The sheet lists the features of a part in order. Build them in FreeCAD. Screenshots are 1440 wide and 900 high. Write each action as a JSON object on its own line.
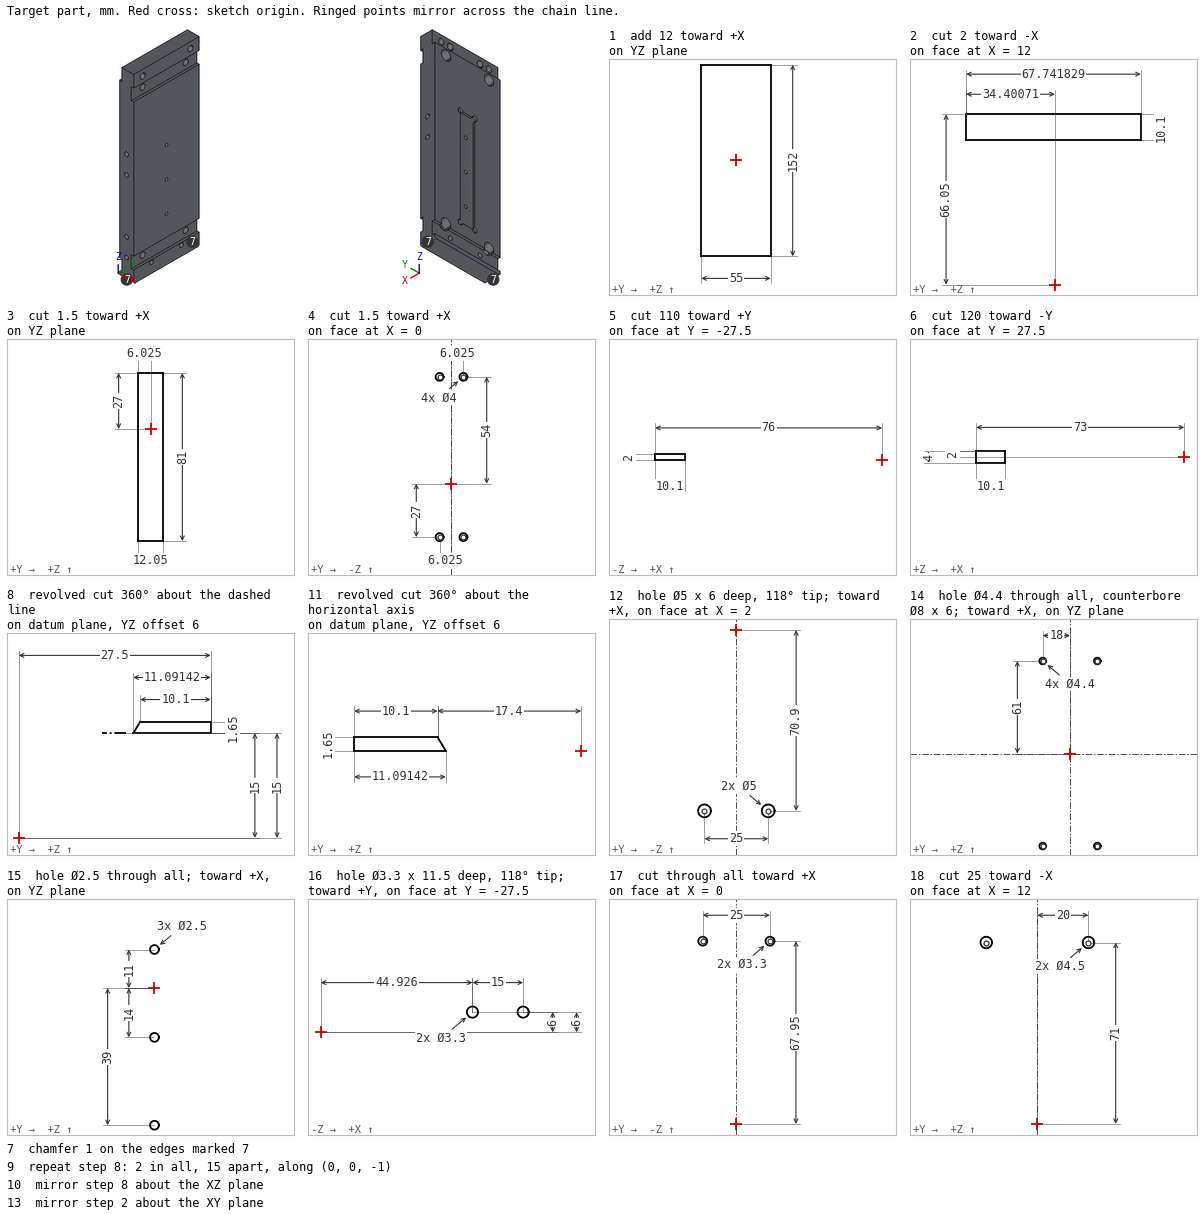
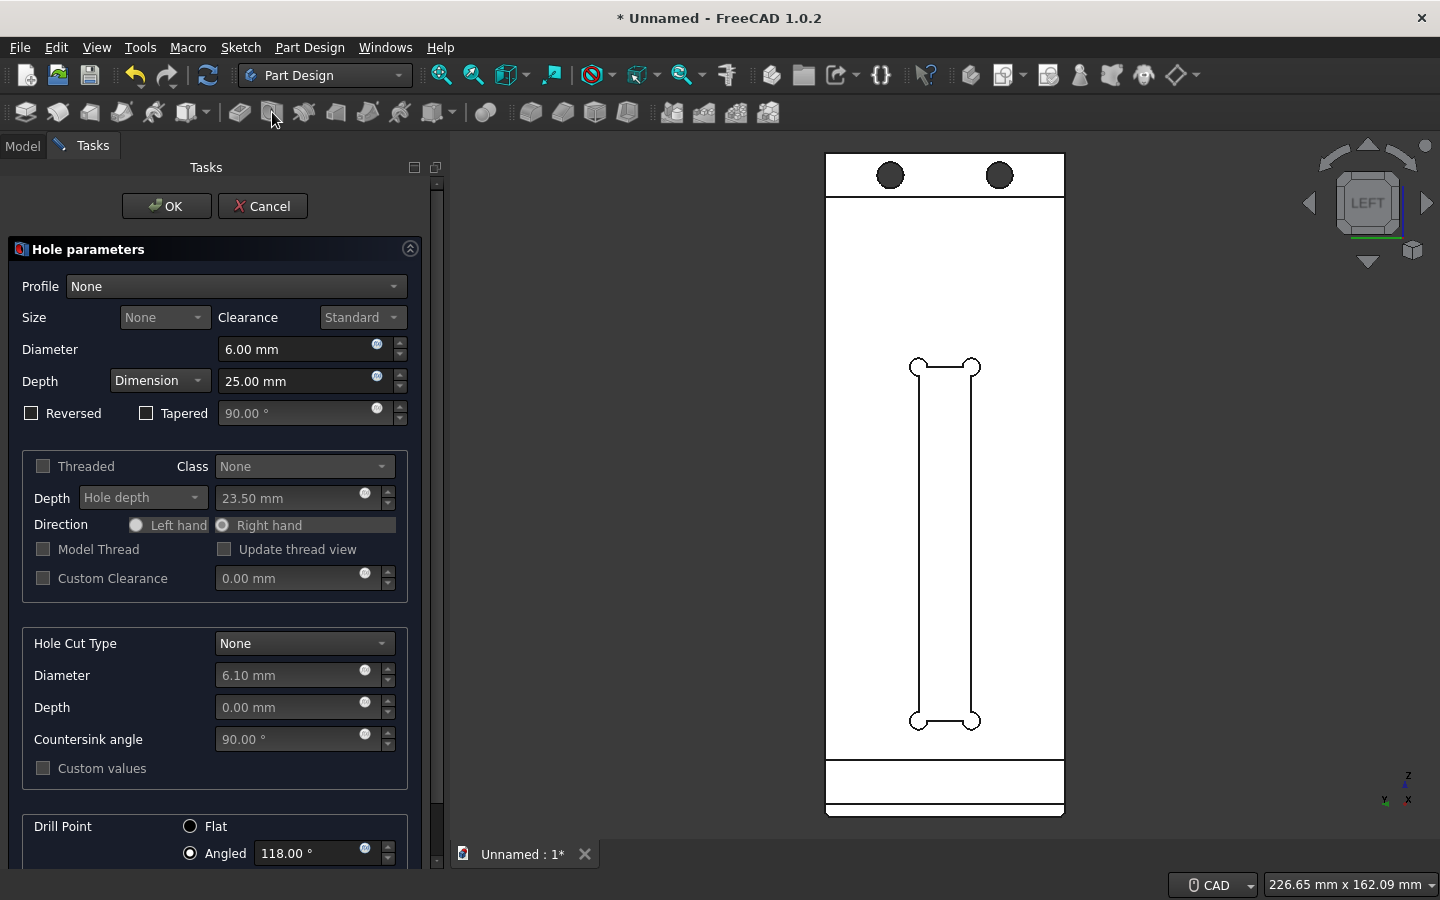
{"action": "triple_click", "coordinate": [305, 349]}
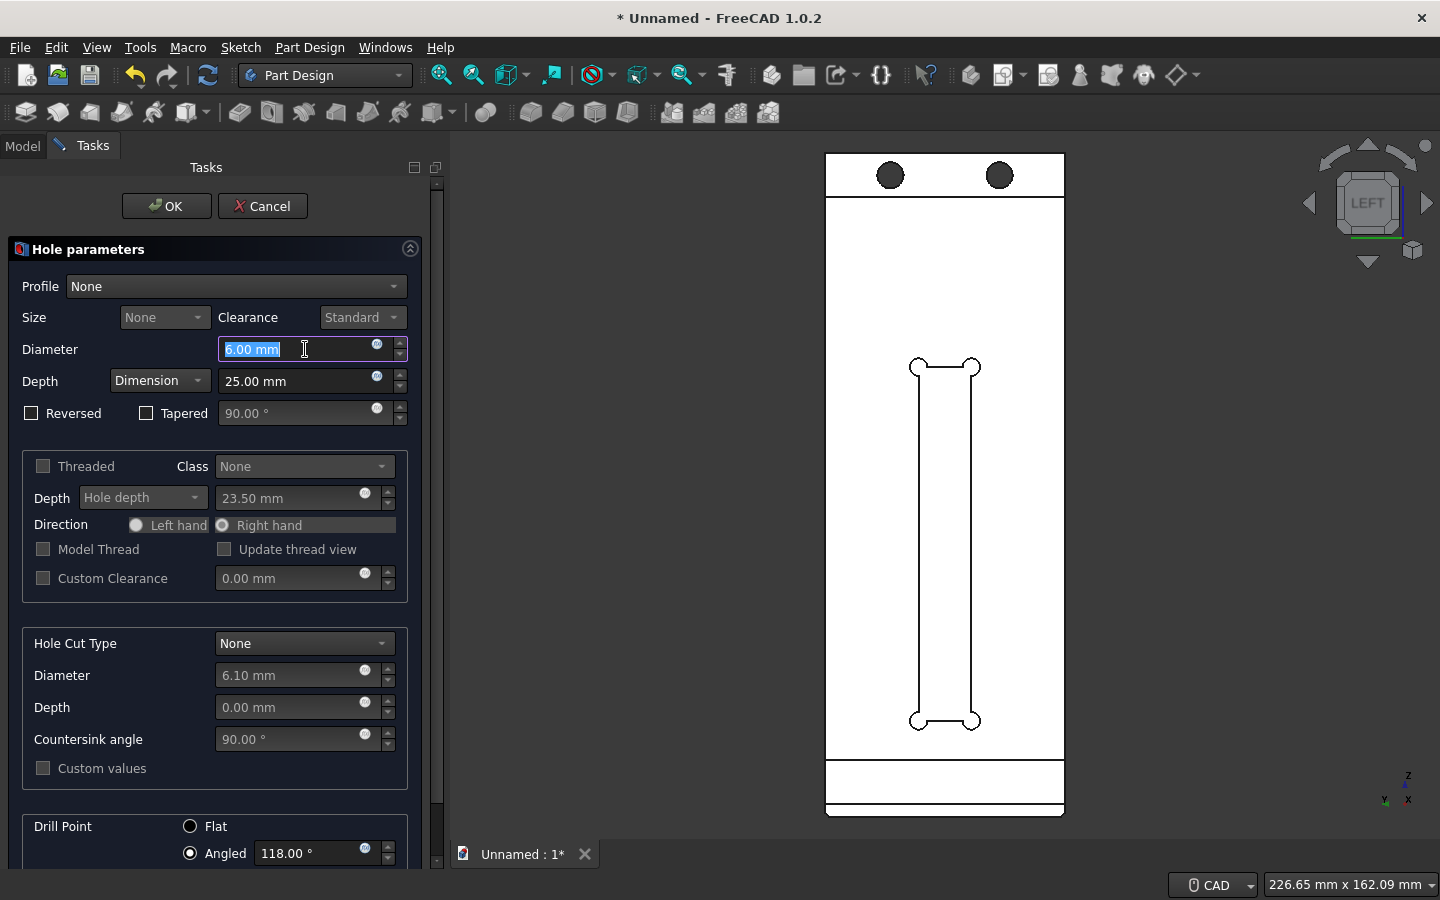
{"action": "type", "text": "5"}
{"action": "key", "text": "Tab"}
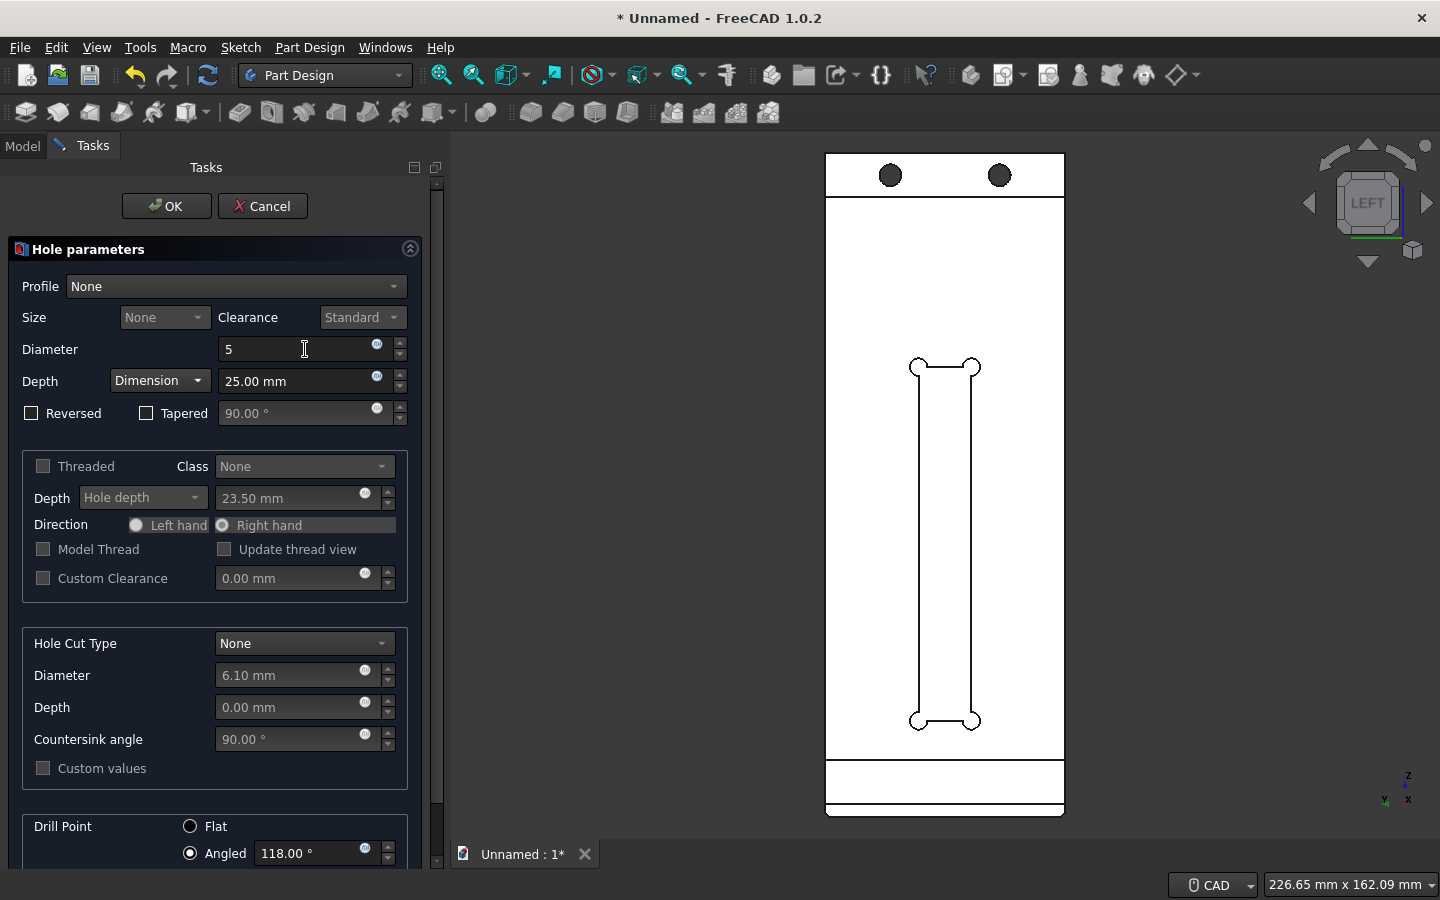
{"action": "triple_click", "coordinate": [305, 381]}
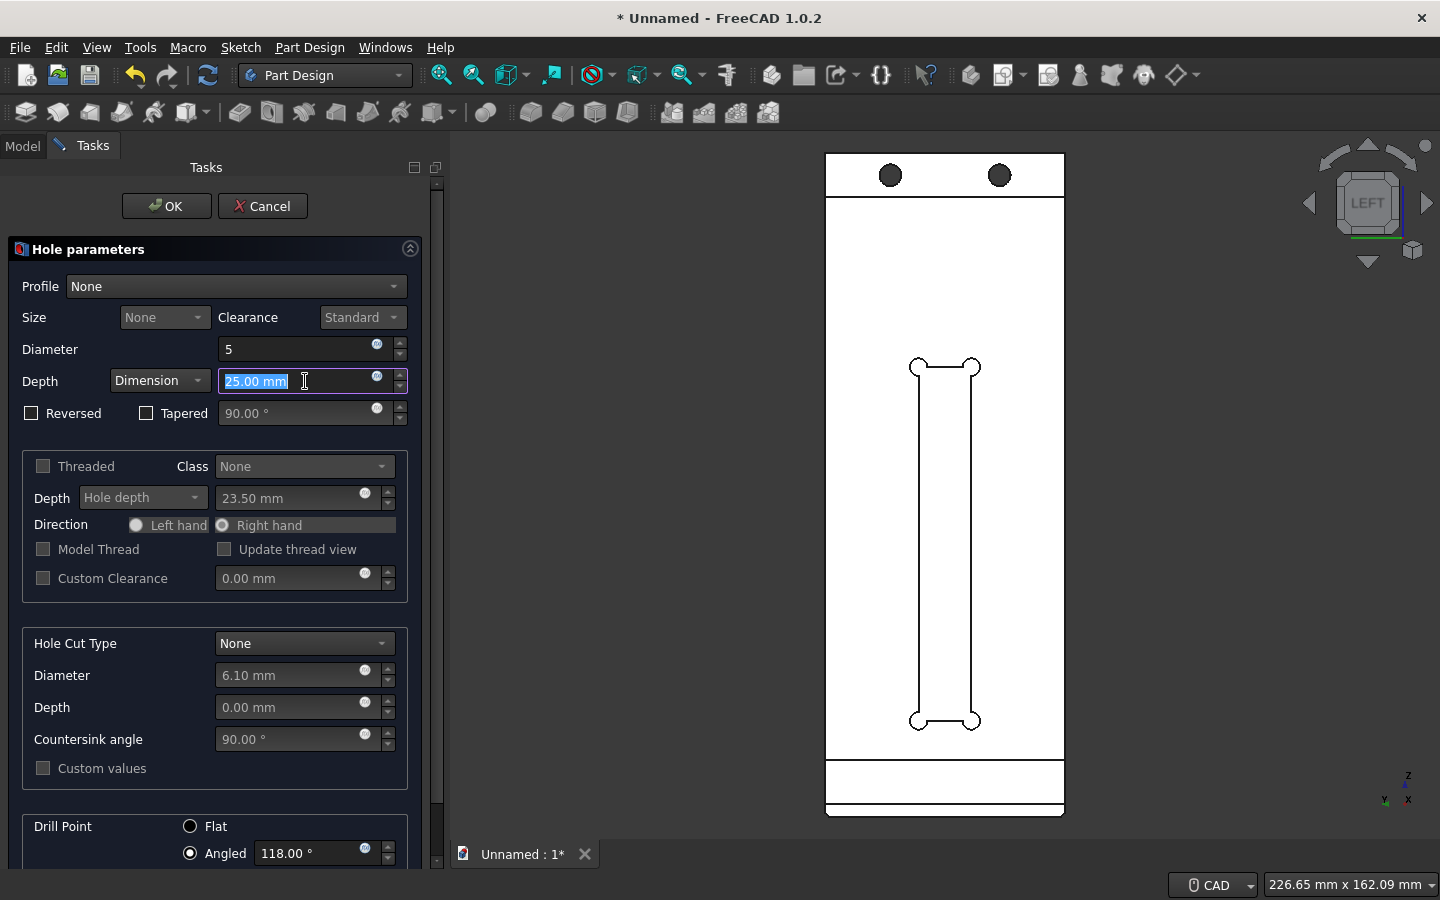
{"action": "type", "text": "6"}
{"action": "key", "text": "Tab"}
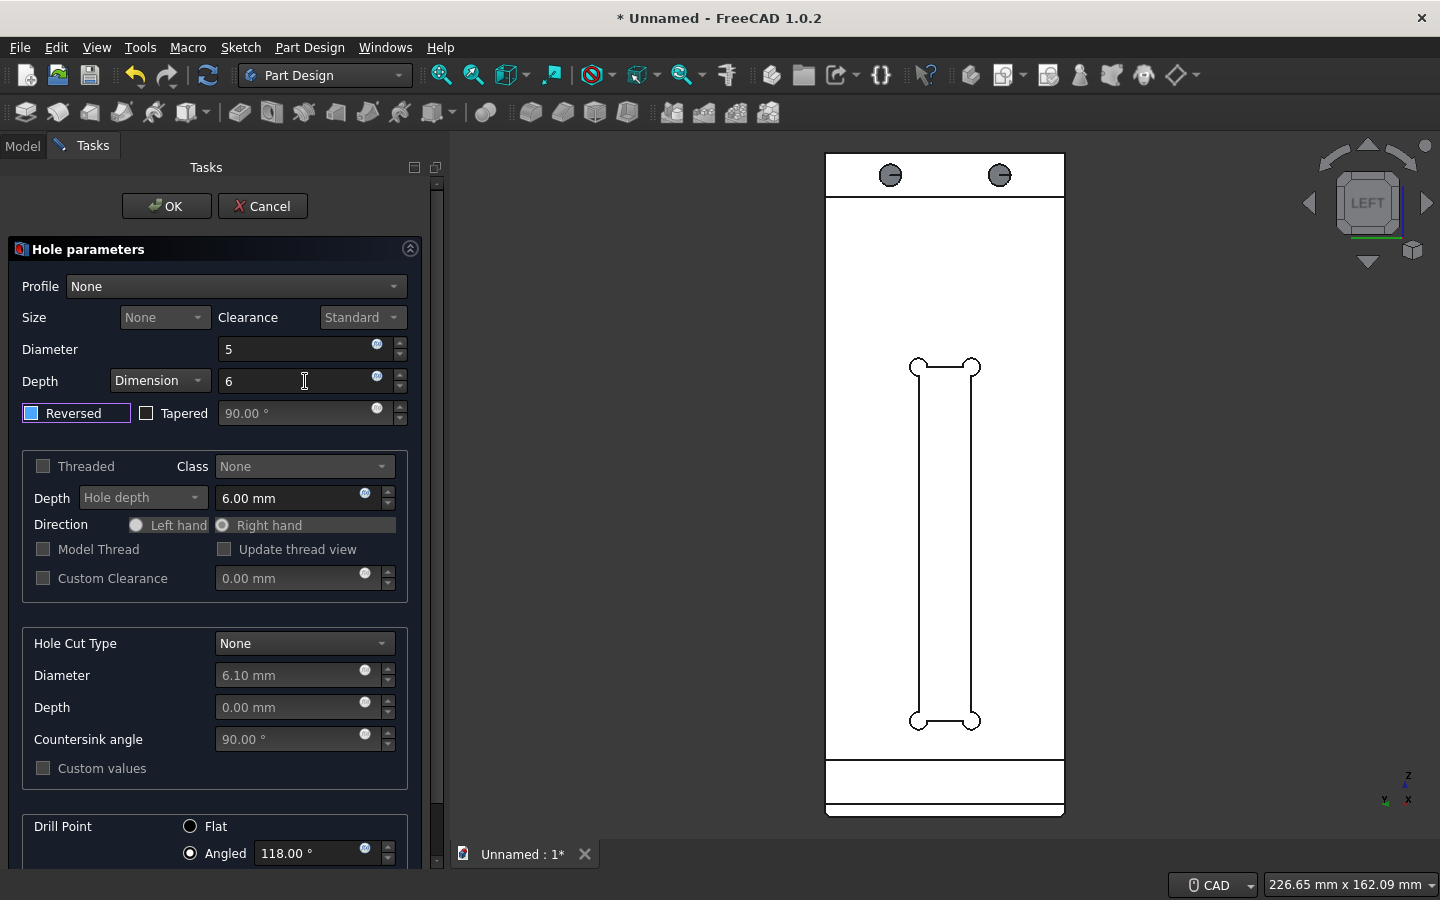
{"action": "left_click", "coordinate": [167, 206]}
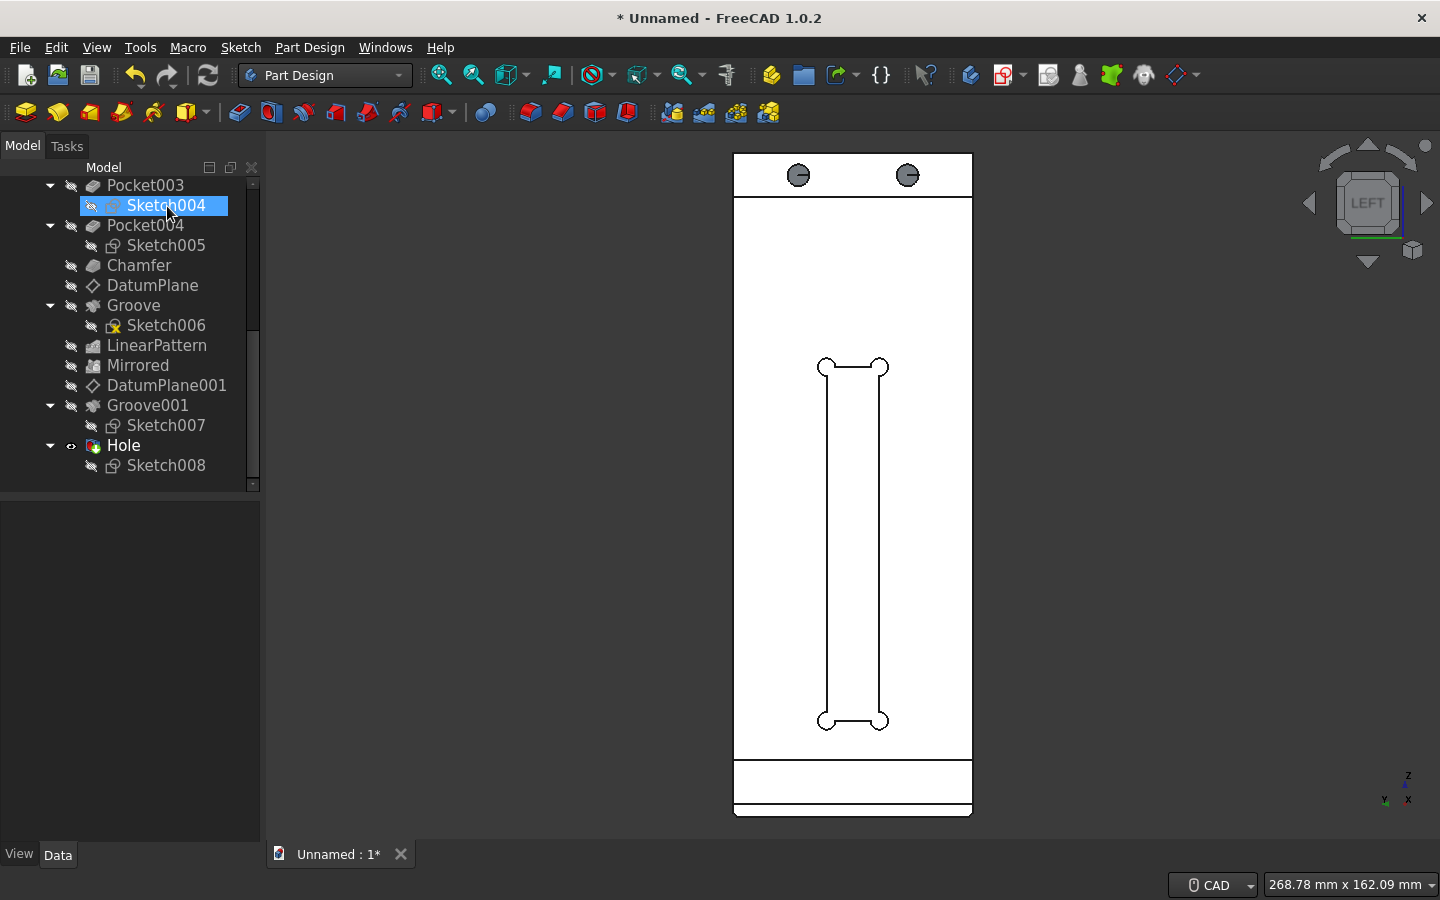
{"action": "scroll", "coordinate": [140, 321], "scroll_direction": "down", "scroll_amount": 3}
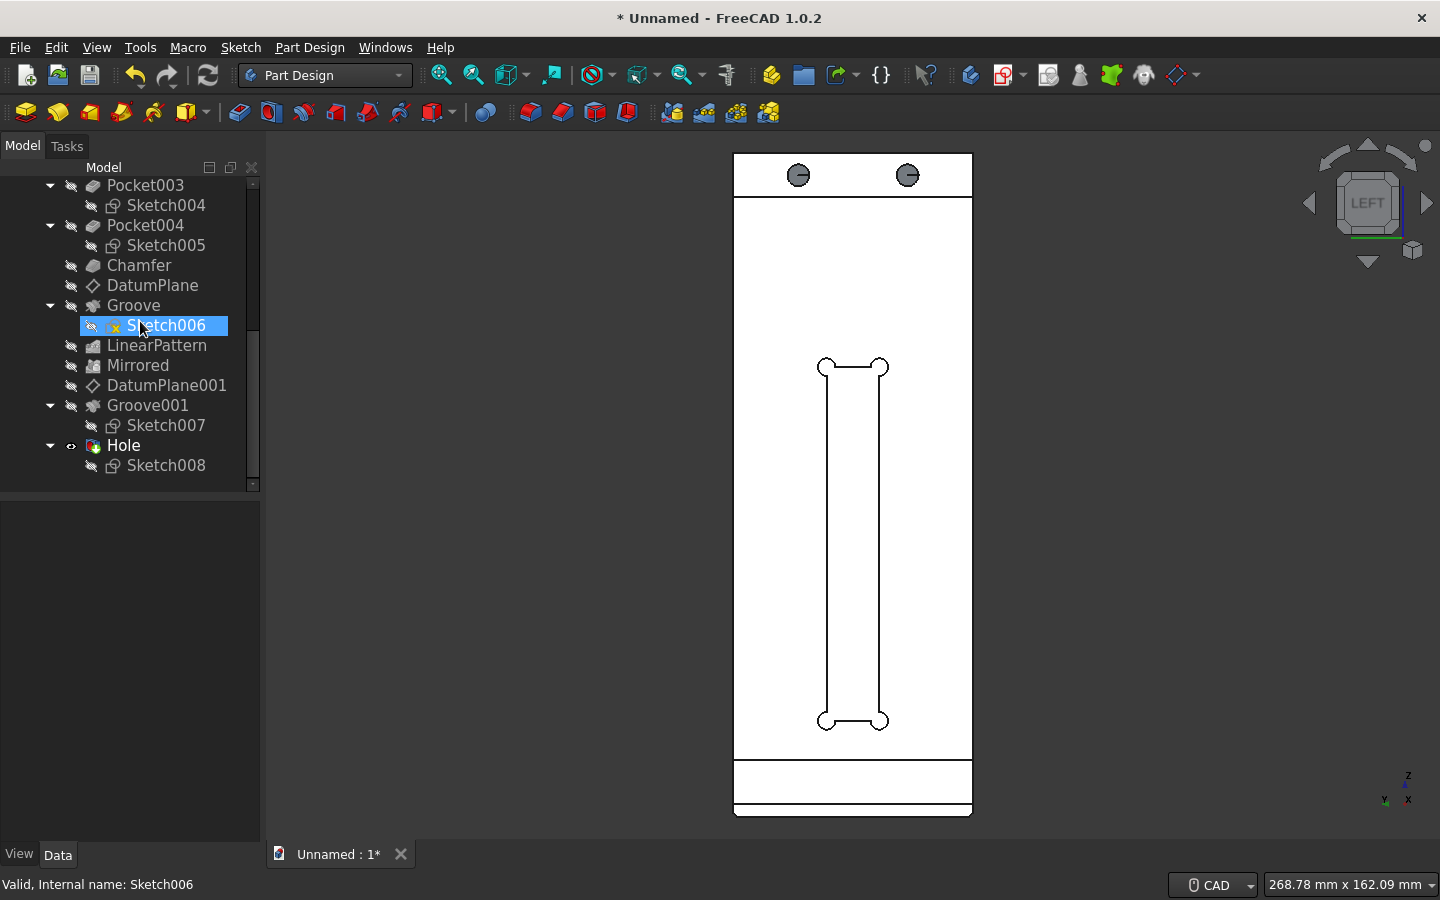
{"action": "scroll", "coordinate": [140, 321], "scroll_direction": "up", "scroll_amount": 15}